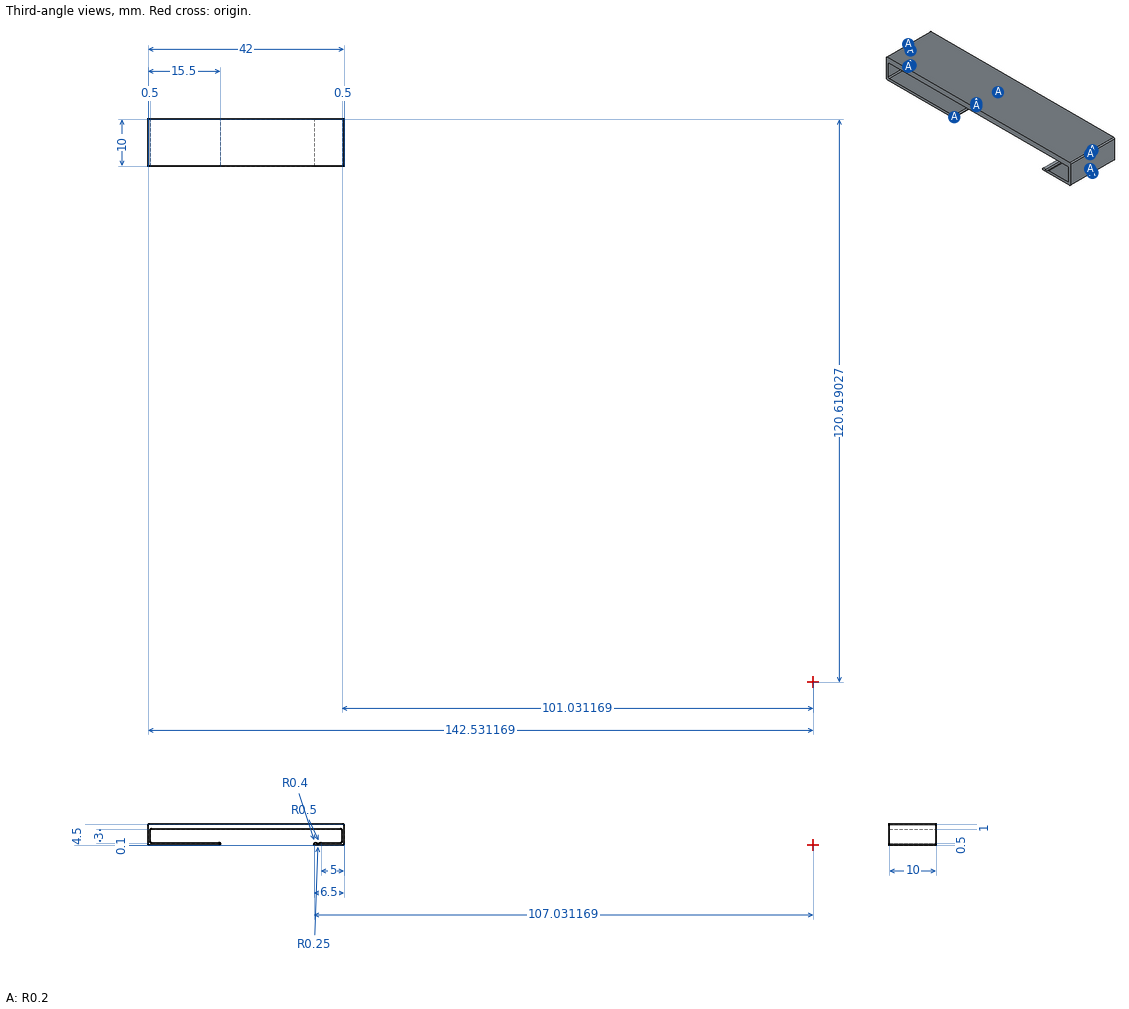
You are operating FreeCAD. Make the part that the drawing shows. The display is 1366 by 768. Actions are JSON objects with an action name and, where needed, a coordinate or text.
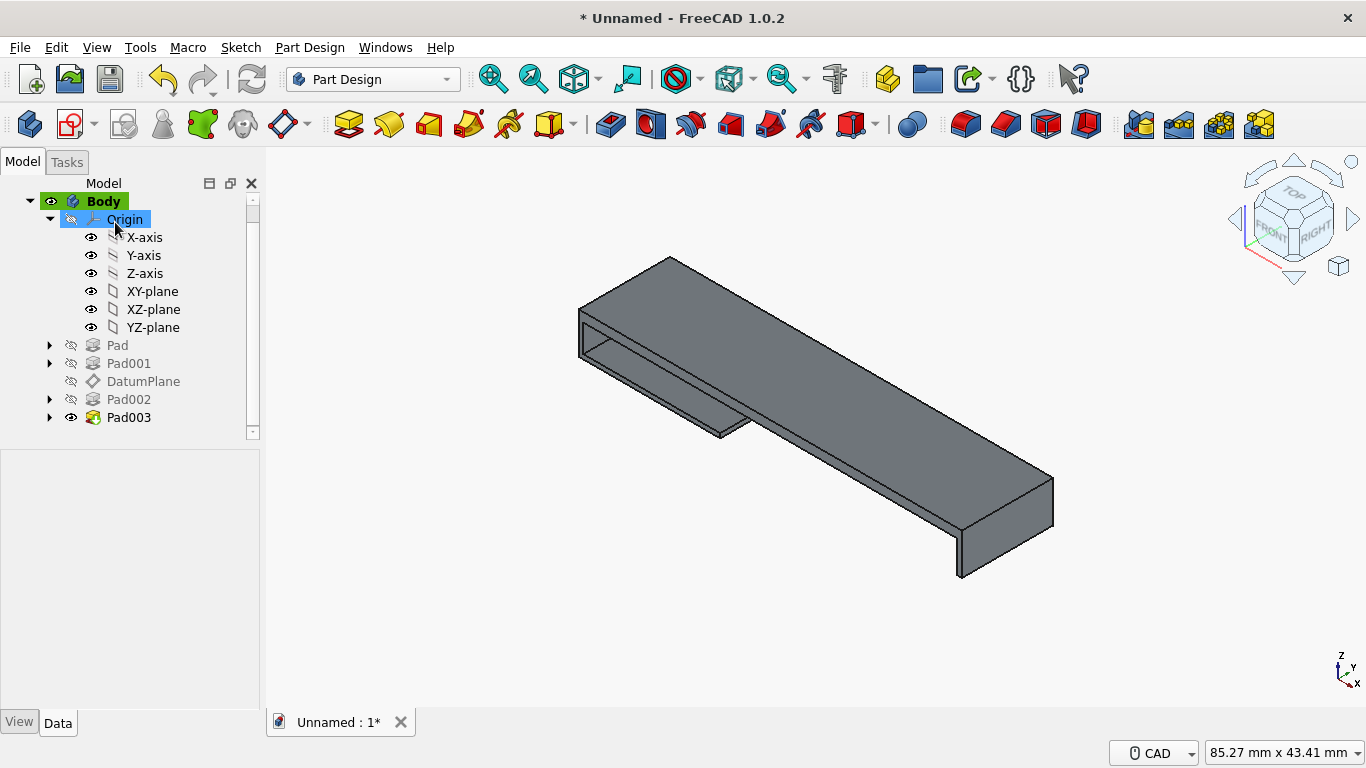
{"action": "scroll", "coordinate": [935, 517], "scroll_direction": "up", "scroll_amount": 6}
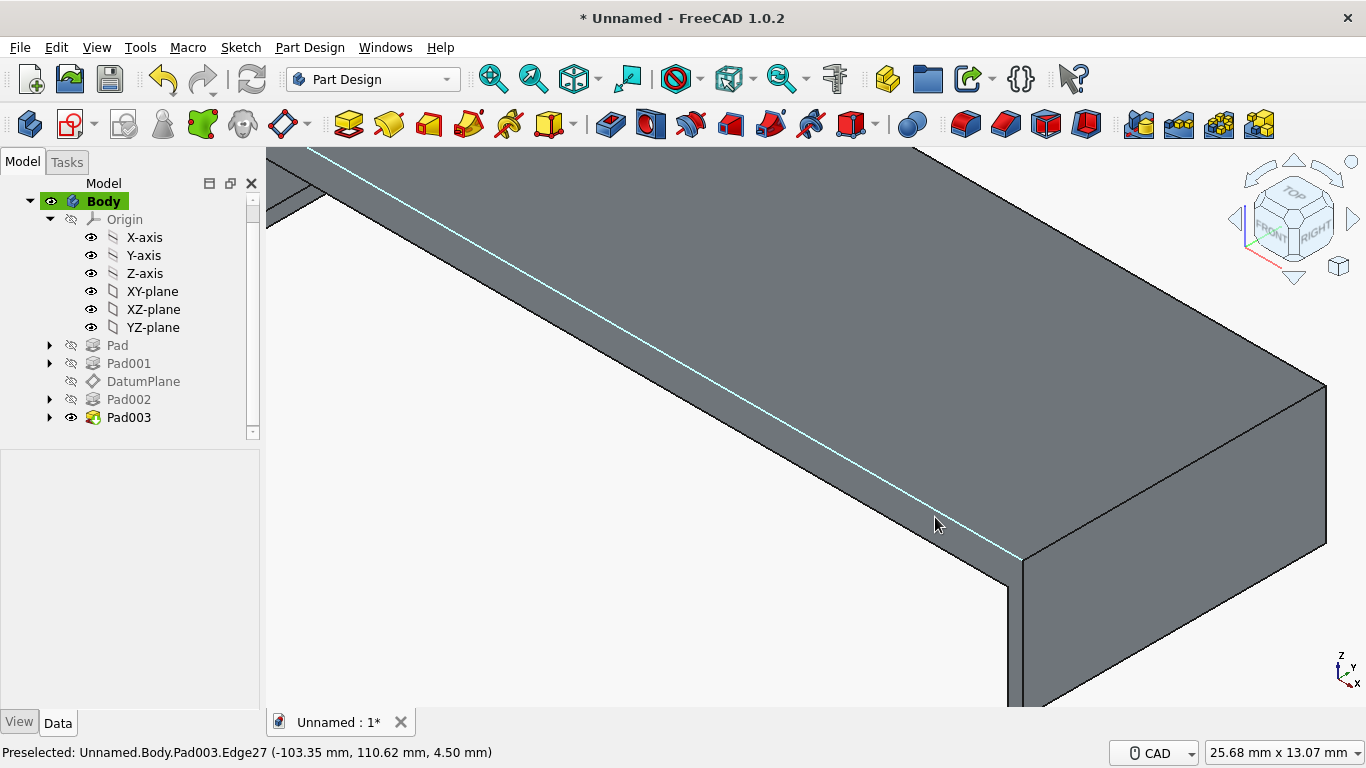
{"action": "left_click", "coordinate": [932, 518]}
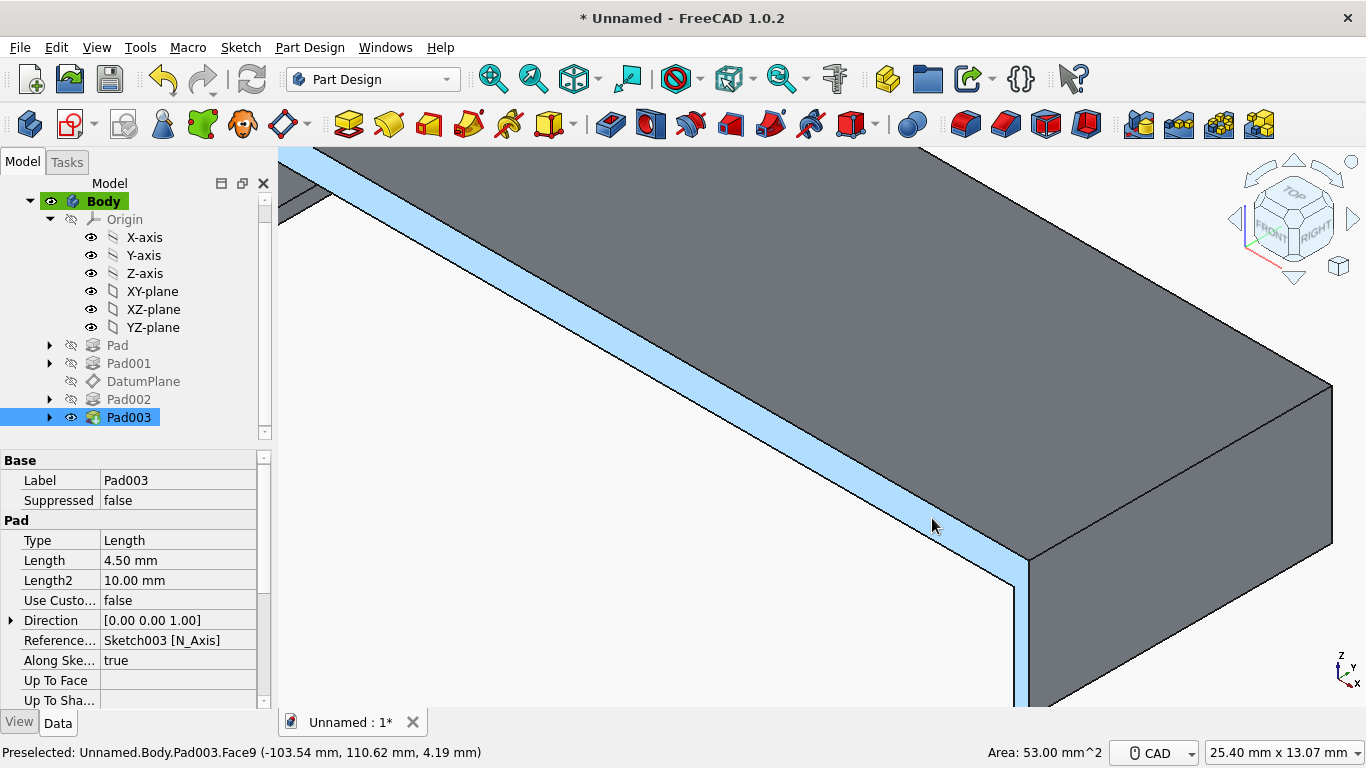
{"action": "left_click", "coordinate": [70, 124]}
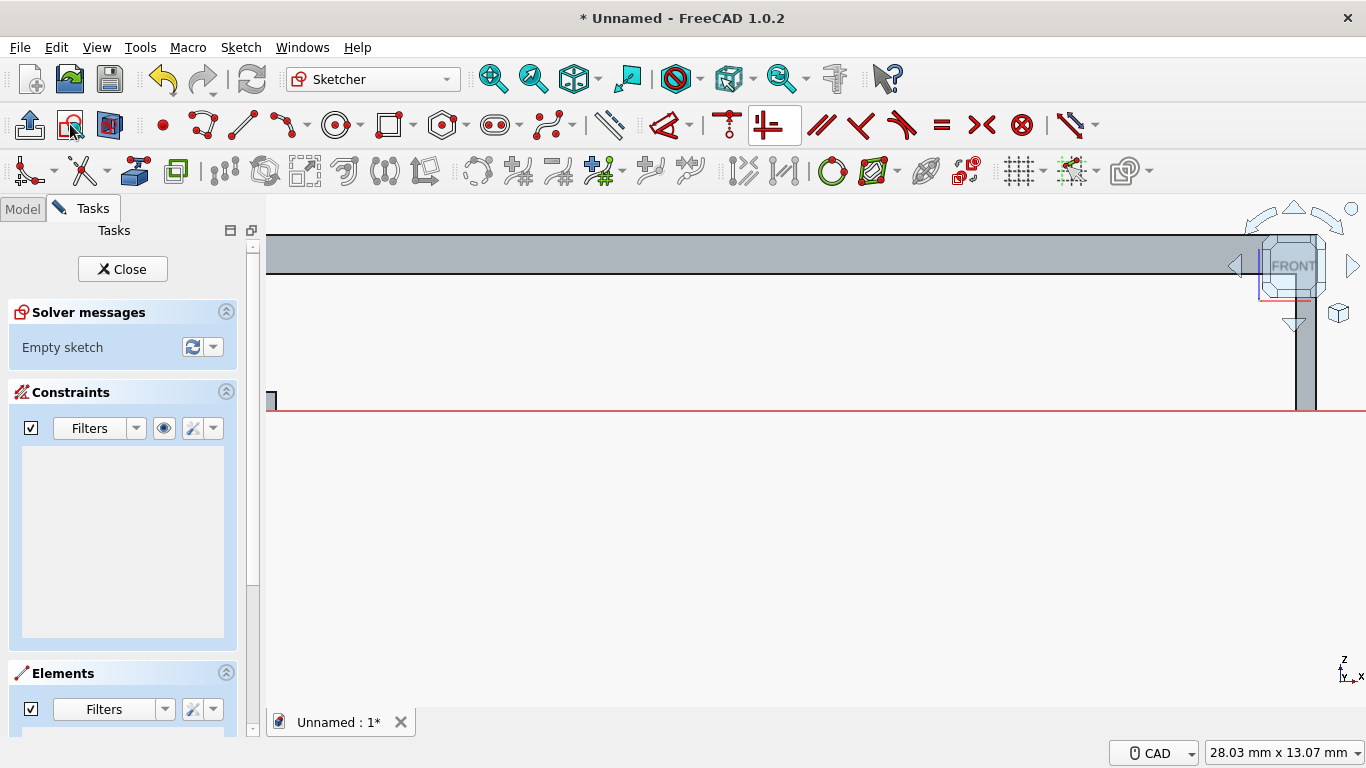
{"action": "scroll", "coordinate": [748, 450], "scroll_direction": "down", "scroll_amount": 5}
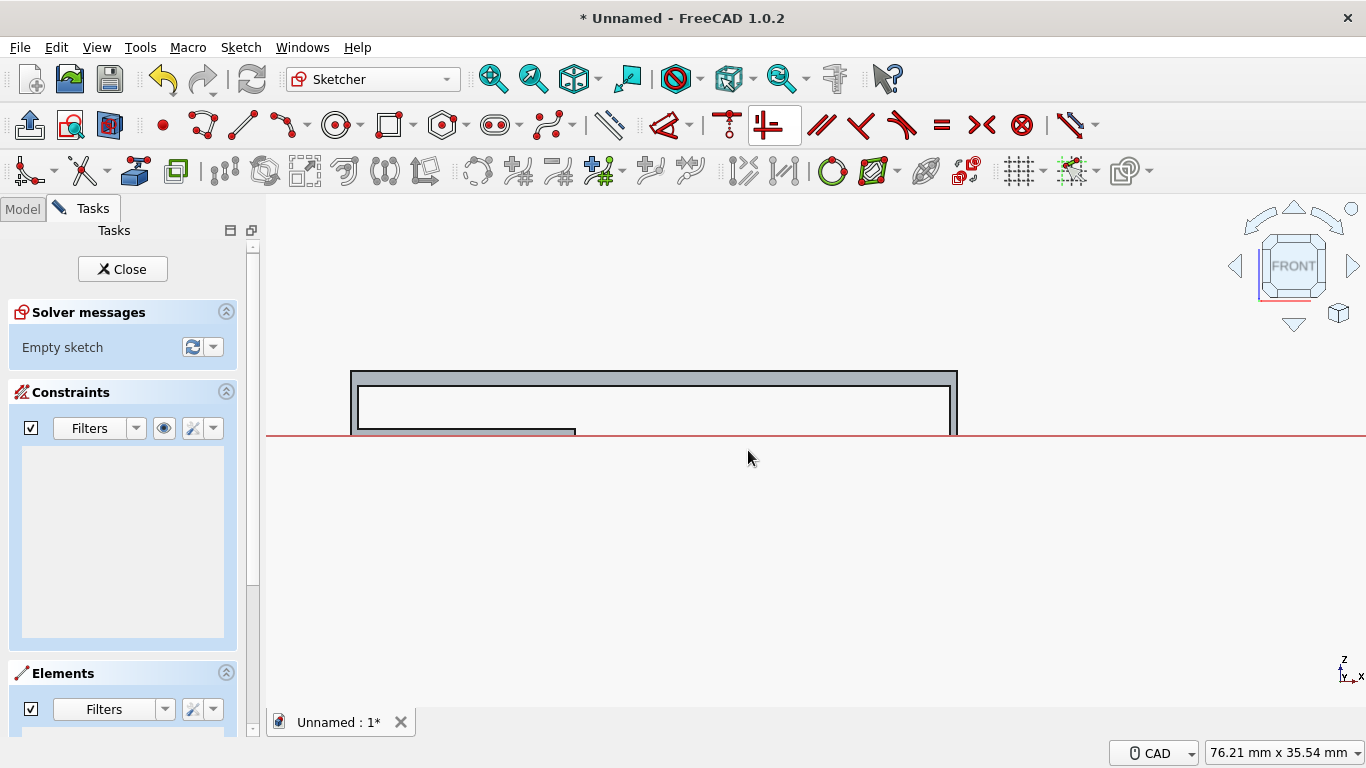
{"action": "scroll", "coordinate": [936, 430], "scroll_direction": "up", "scroll_amount": 10}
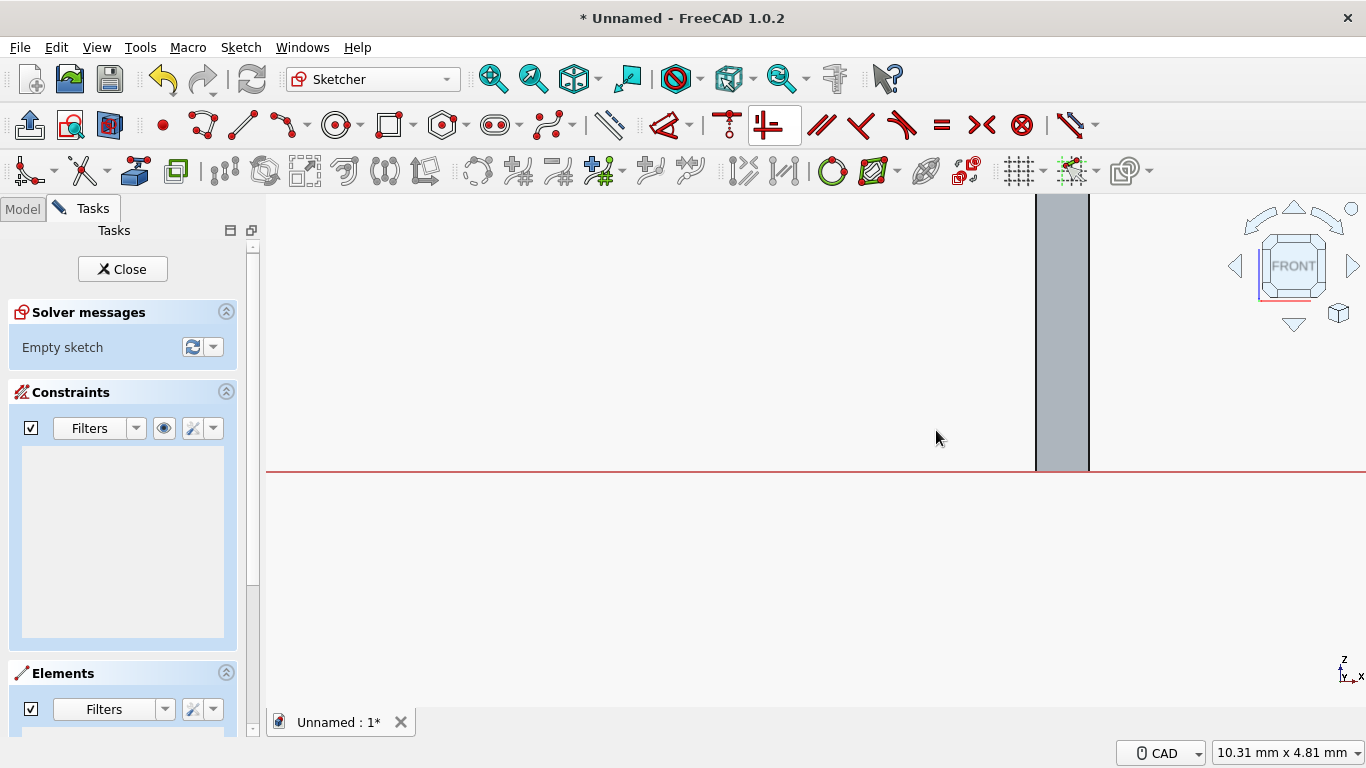
{"action": "left_click", "coordinate": [204, 126]}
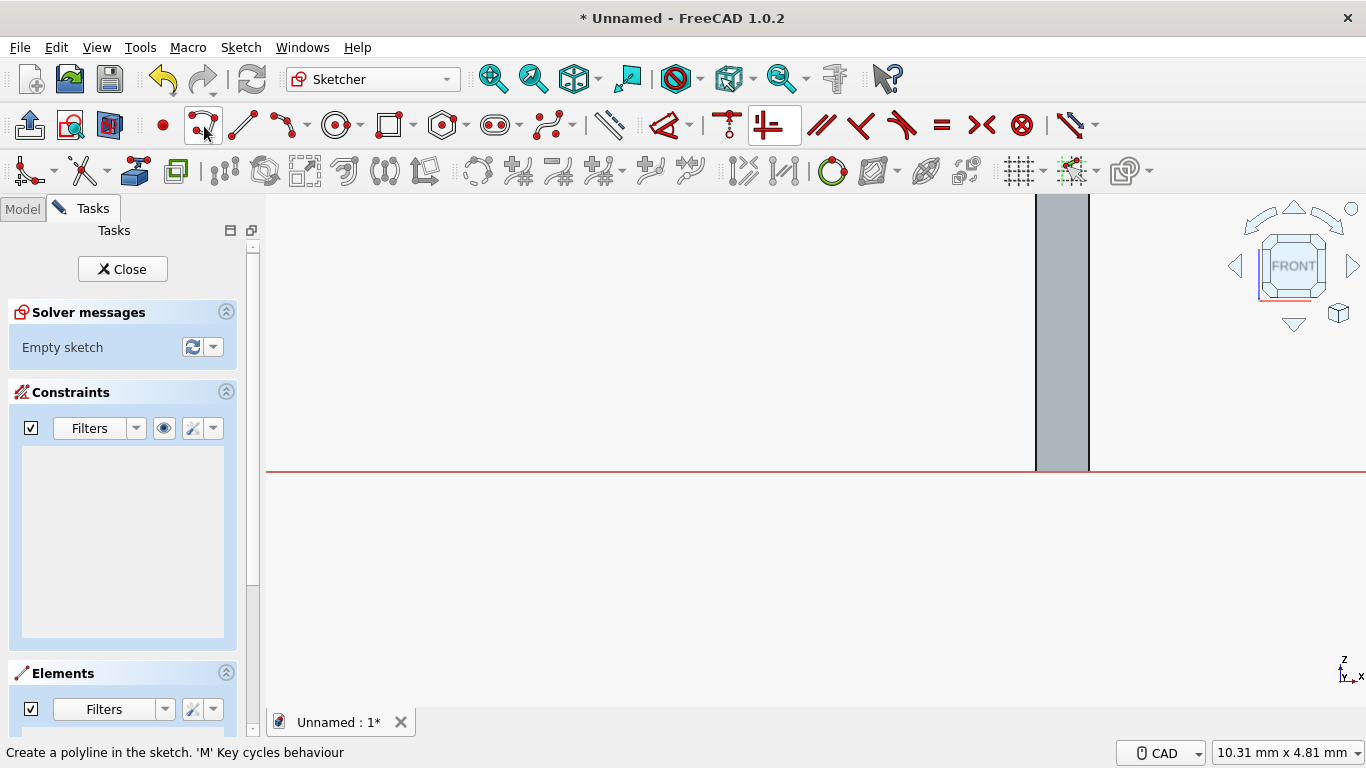
{"action": "scroll", "coordinate": [396, 461], "scroll_direction": "up", "scroll_amount": 2}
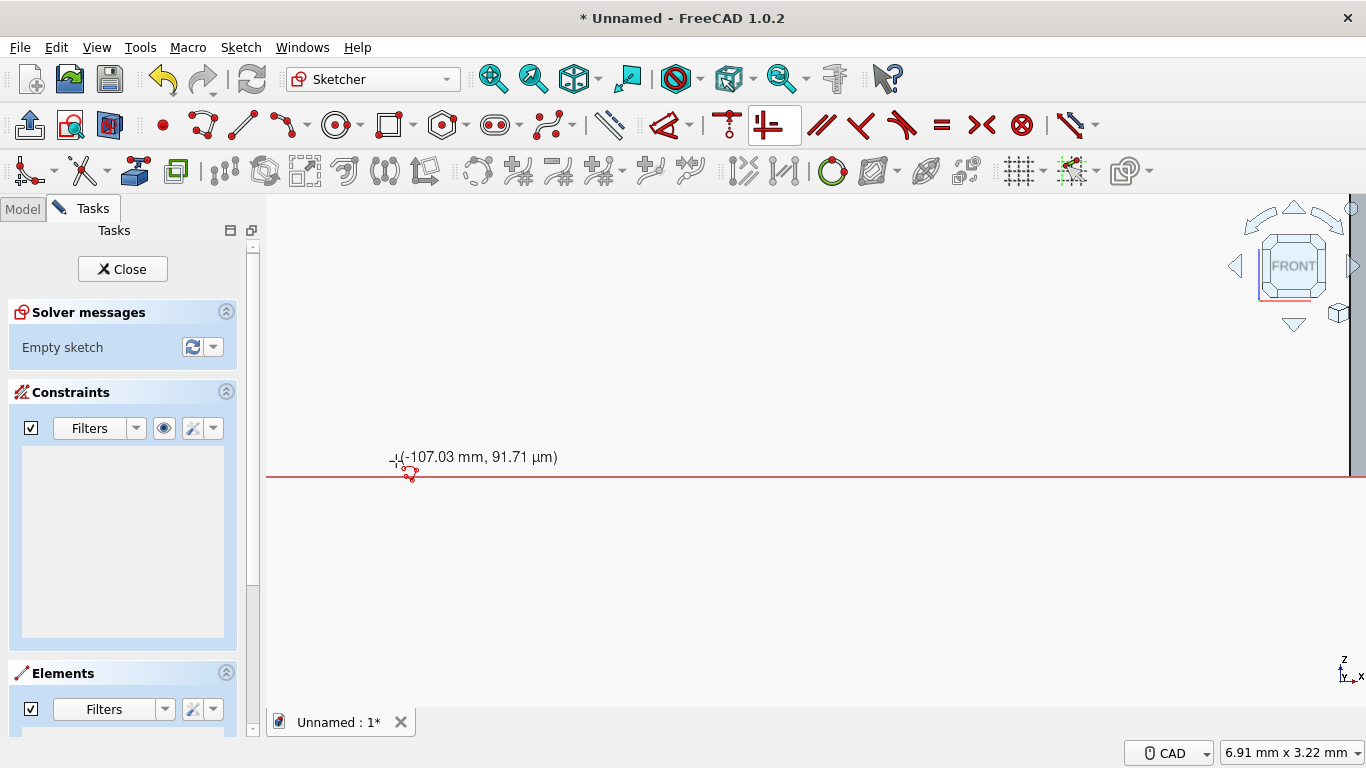
{"action": "left_click", "coordinate": [395, 461]}
{"action": "left_click", "coordinate": [395, 477]}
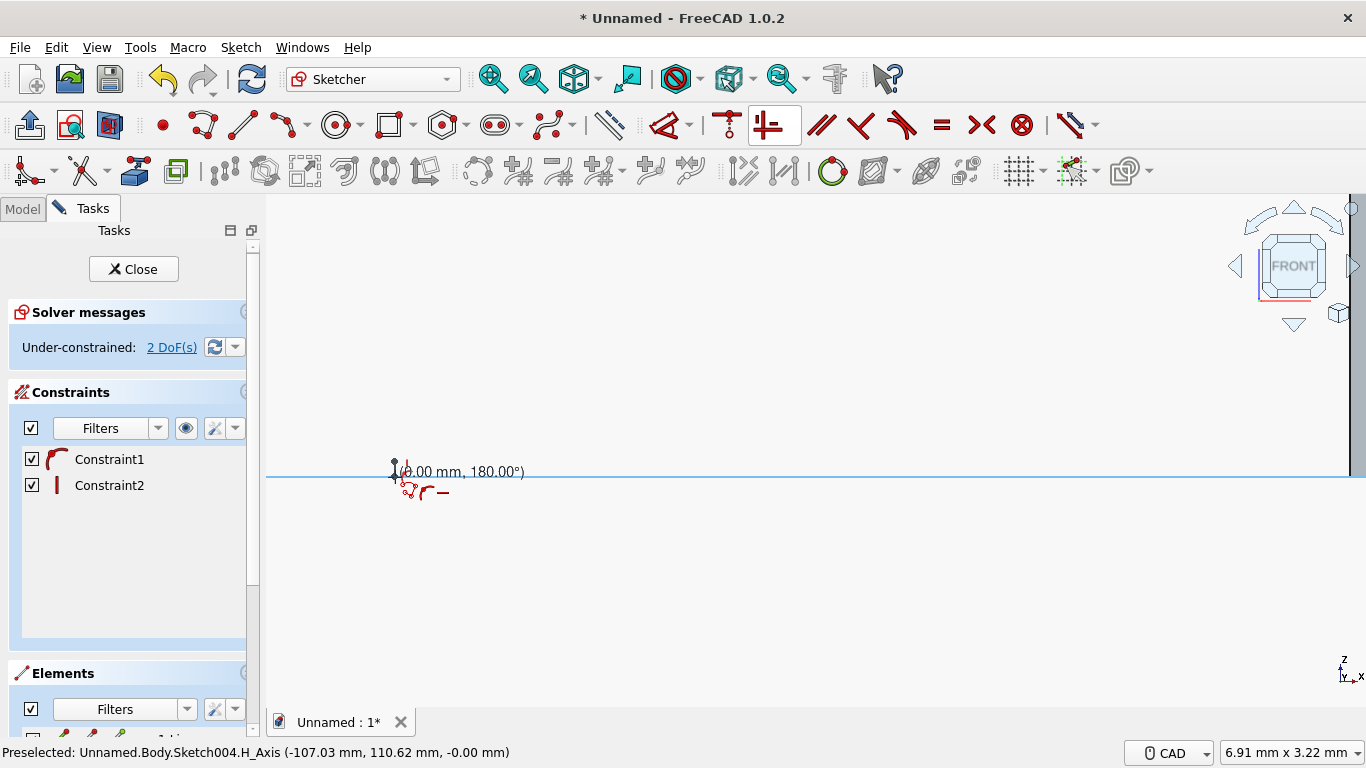
{"action": "scroll", "coordinate": [412, 478], "scroll_direction": "down", "scroll_amount": 2}